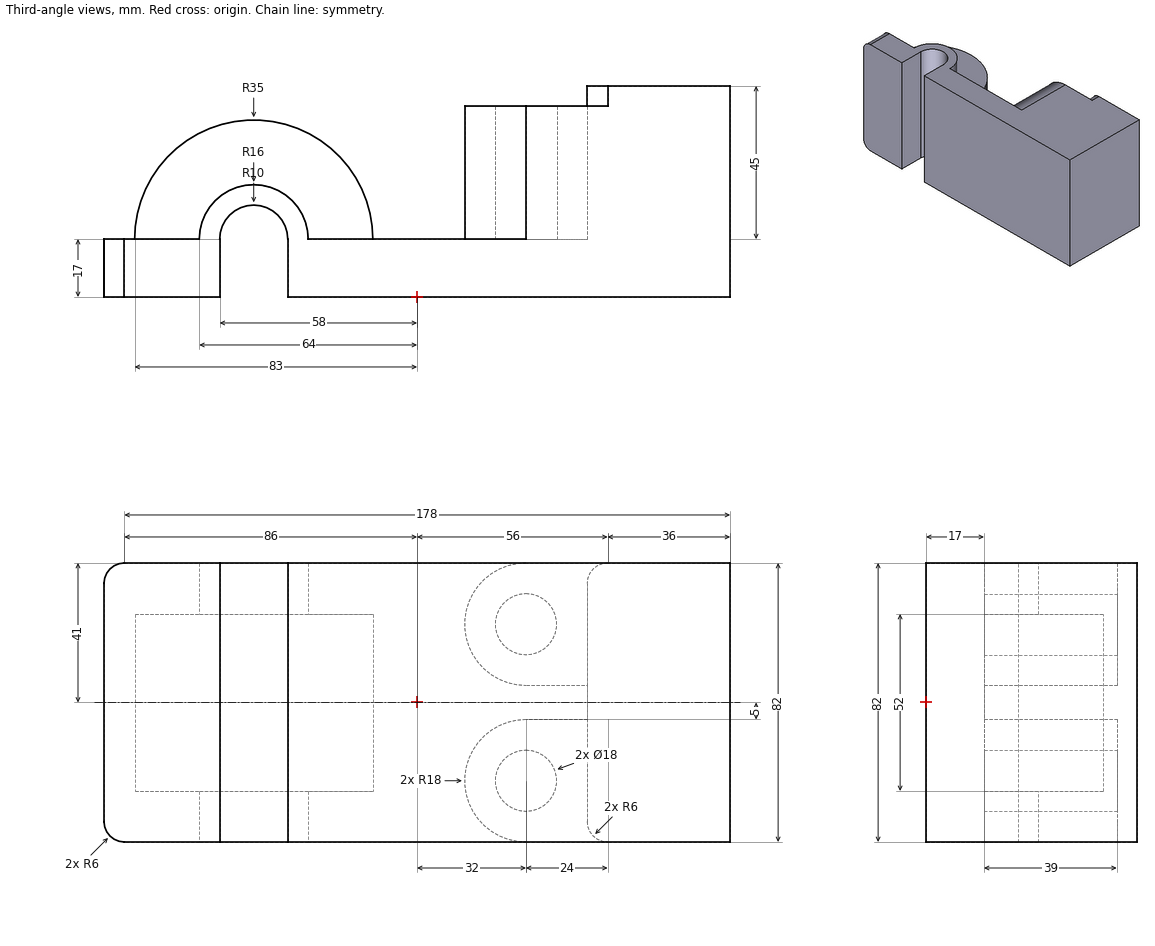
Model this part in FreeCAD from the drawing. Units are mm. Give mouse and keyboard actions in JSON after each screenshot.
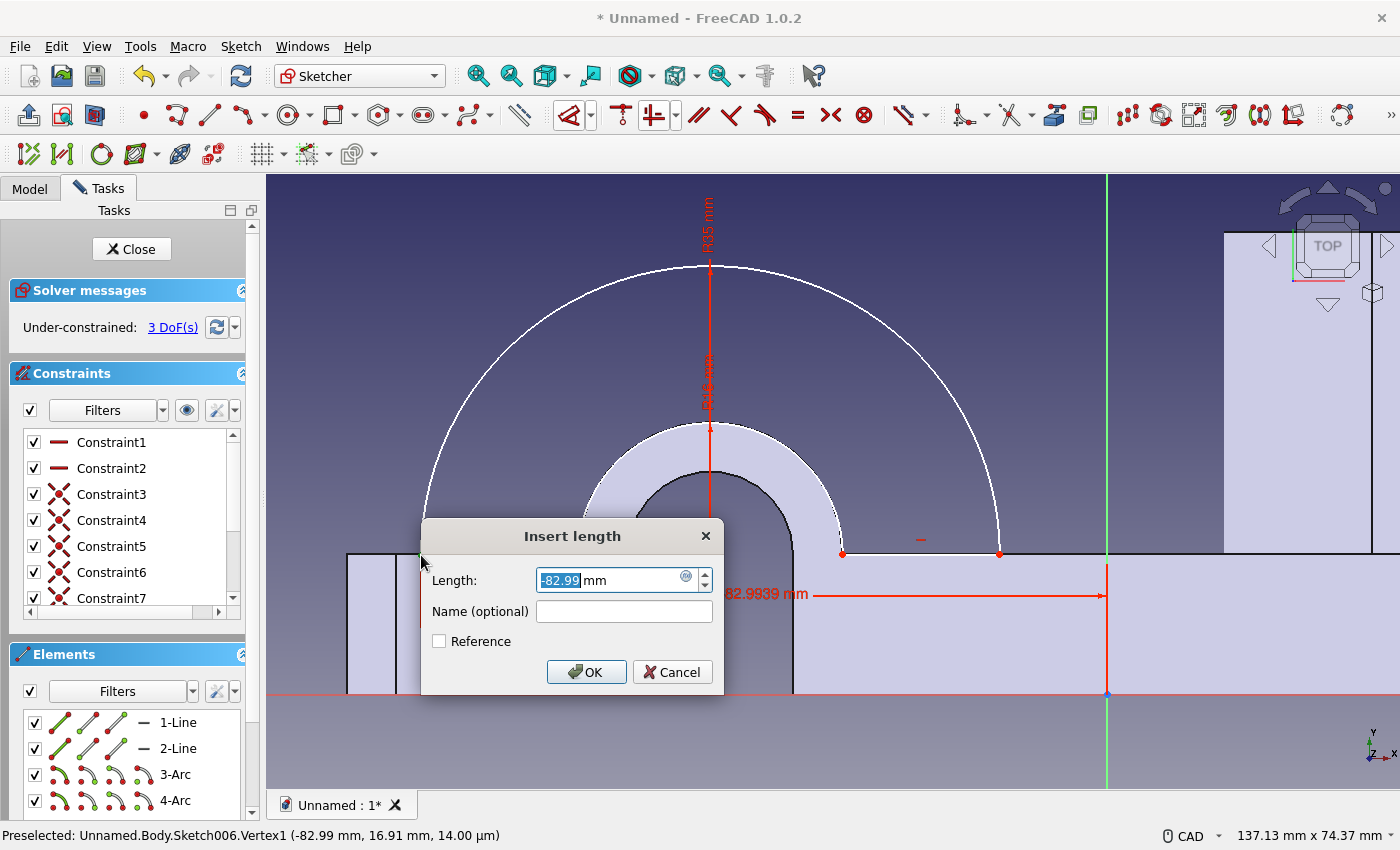
{"action": "type", "text": "-83"}
{"action": "key", "text": "Return"}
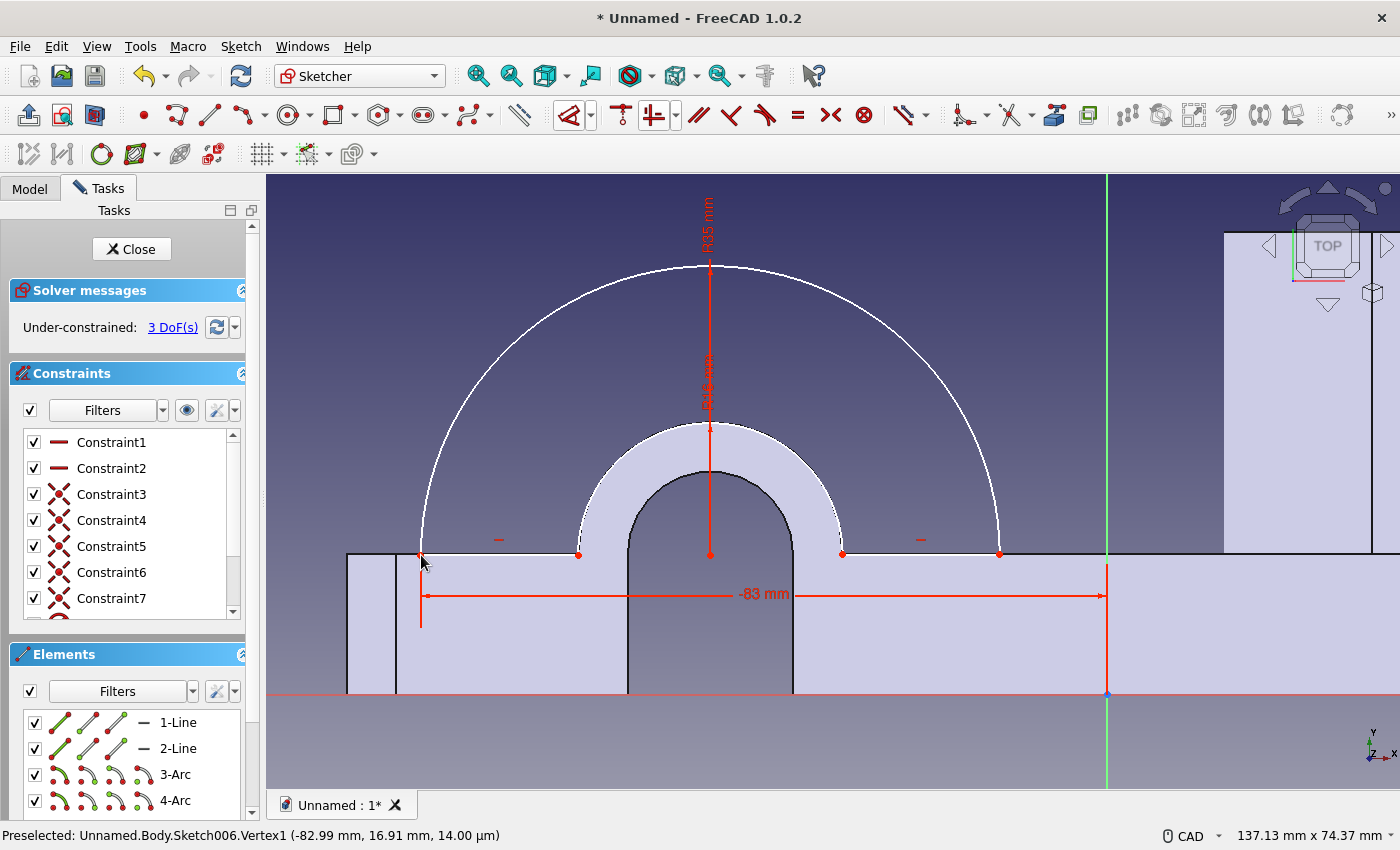
{"action": "left_click", "coordinate": [421, 555]}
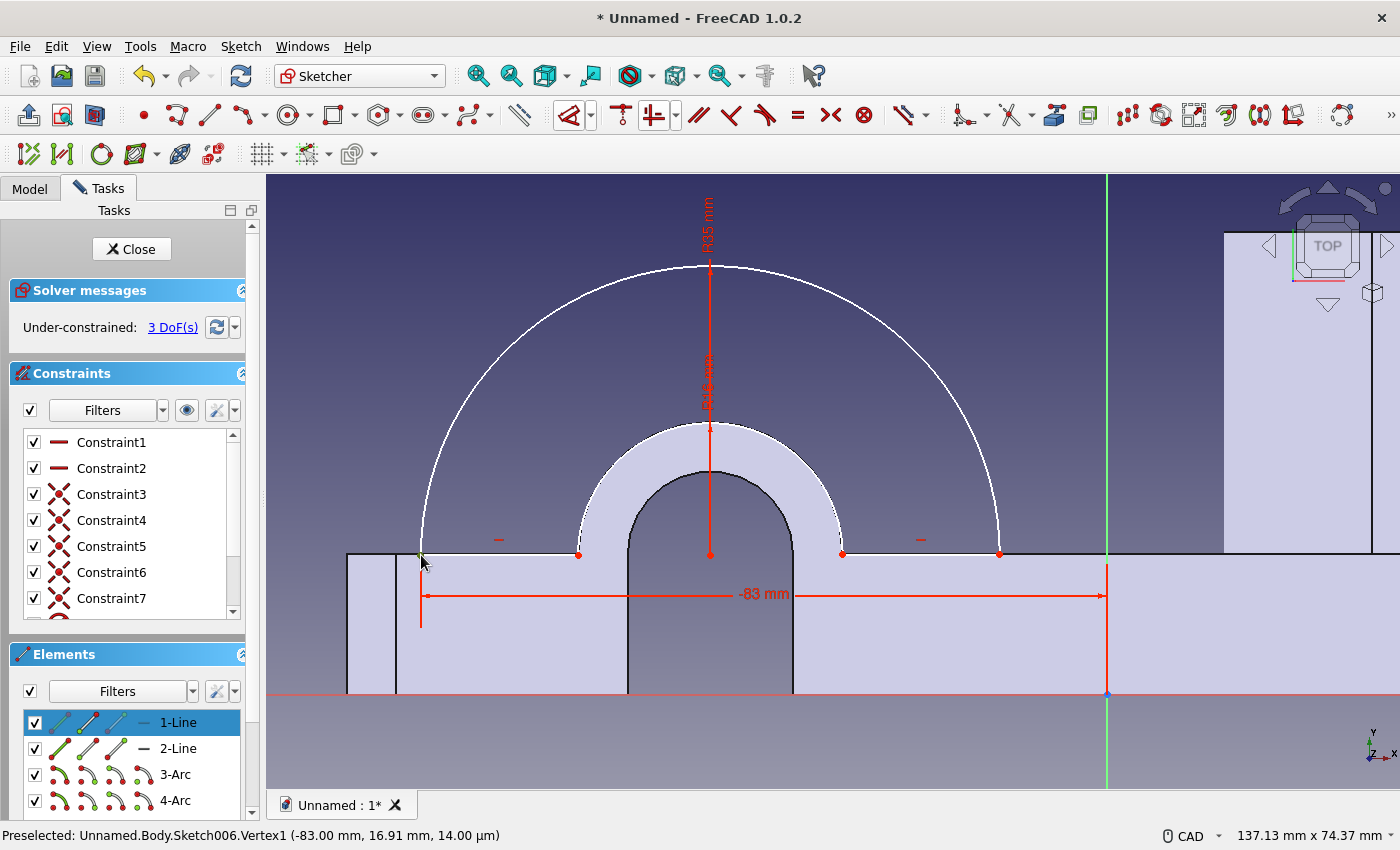
{"action": "left_click", "coordinate": [590, 116]}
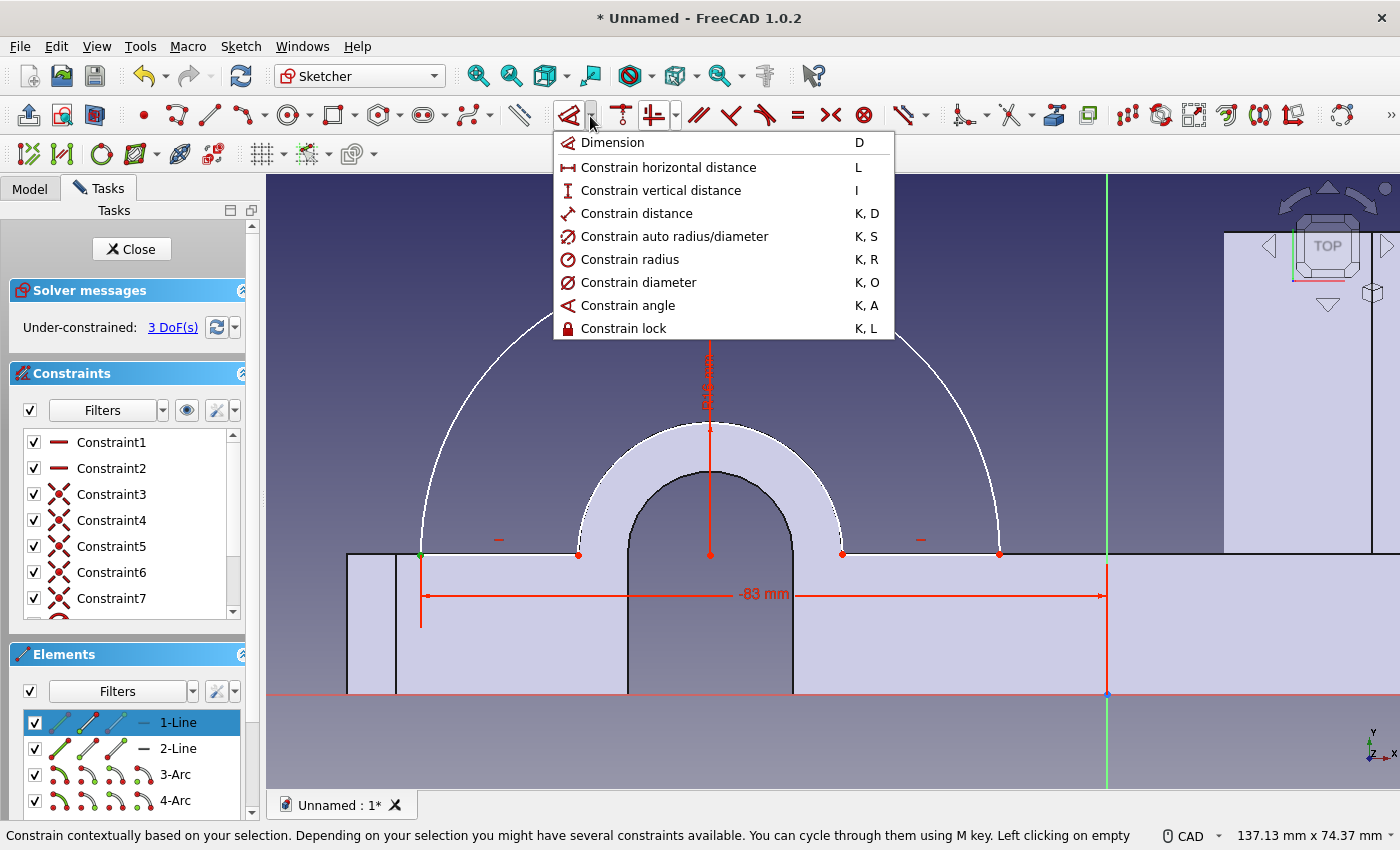
{"action": "left_click", "coordinate": [724, 190]}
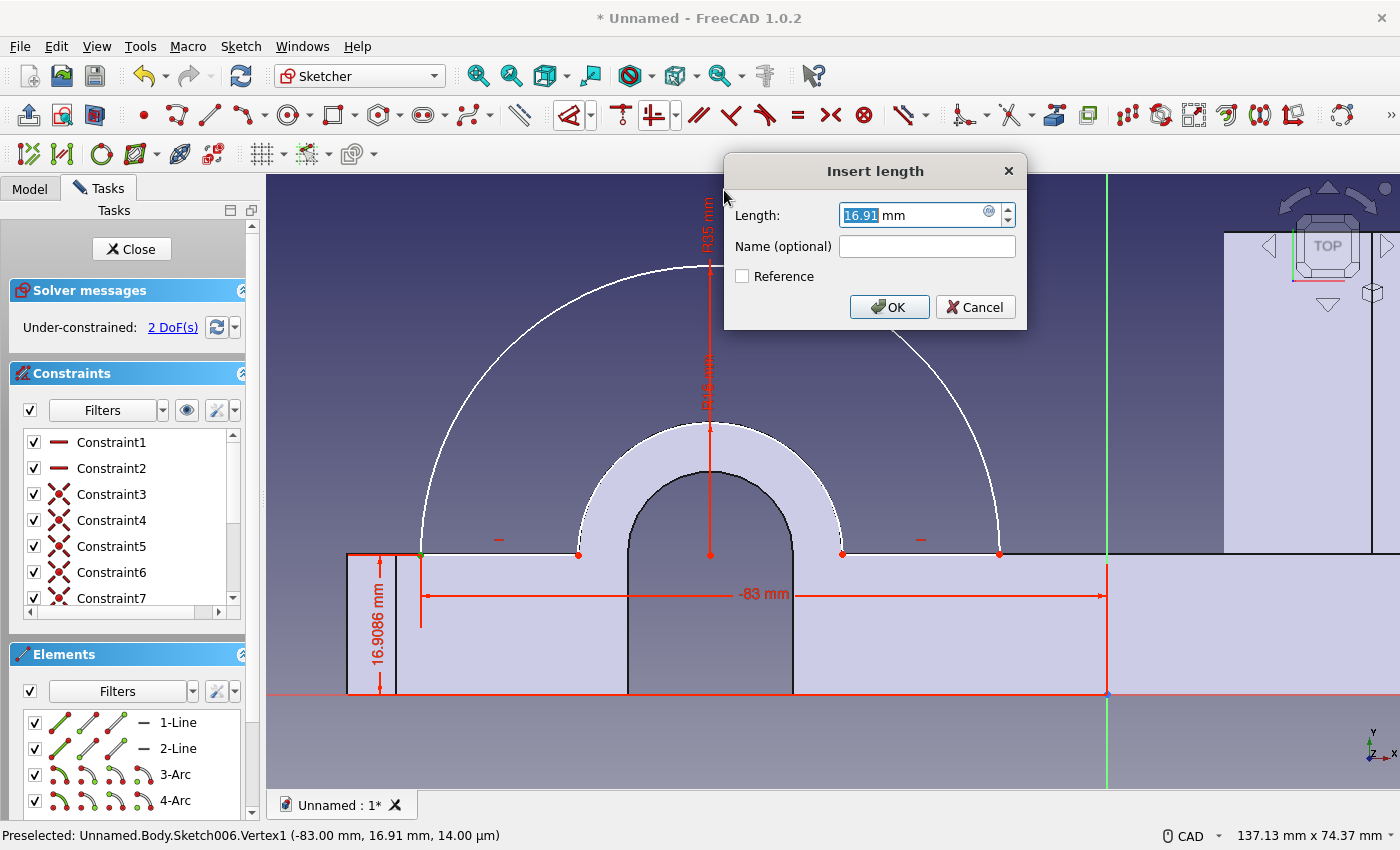
{"action": "type", "text": "17"}
{"action": "key", "text": "Return"}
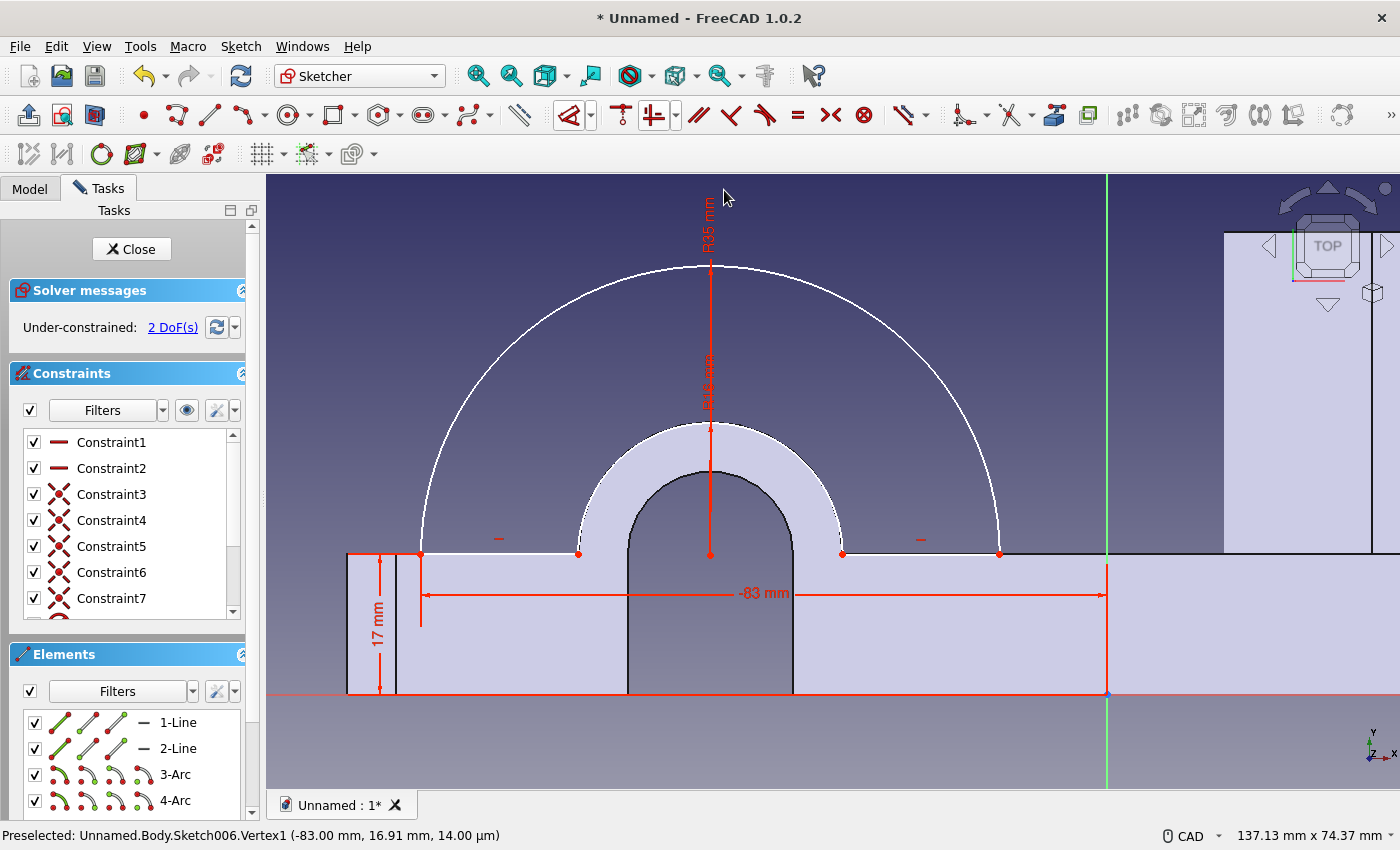
{"action": "left_click", "coordinate": [843, 555]}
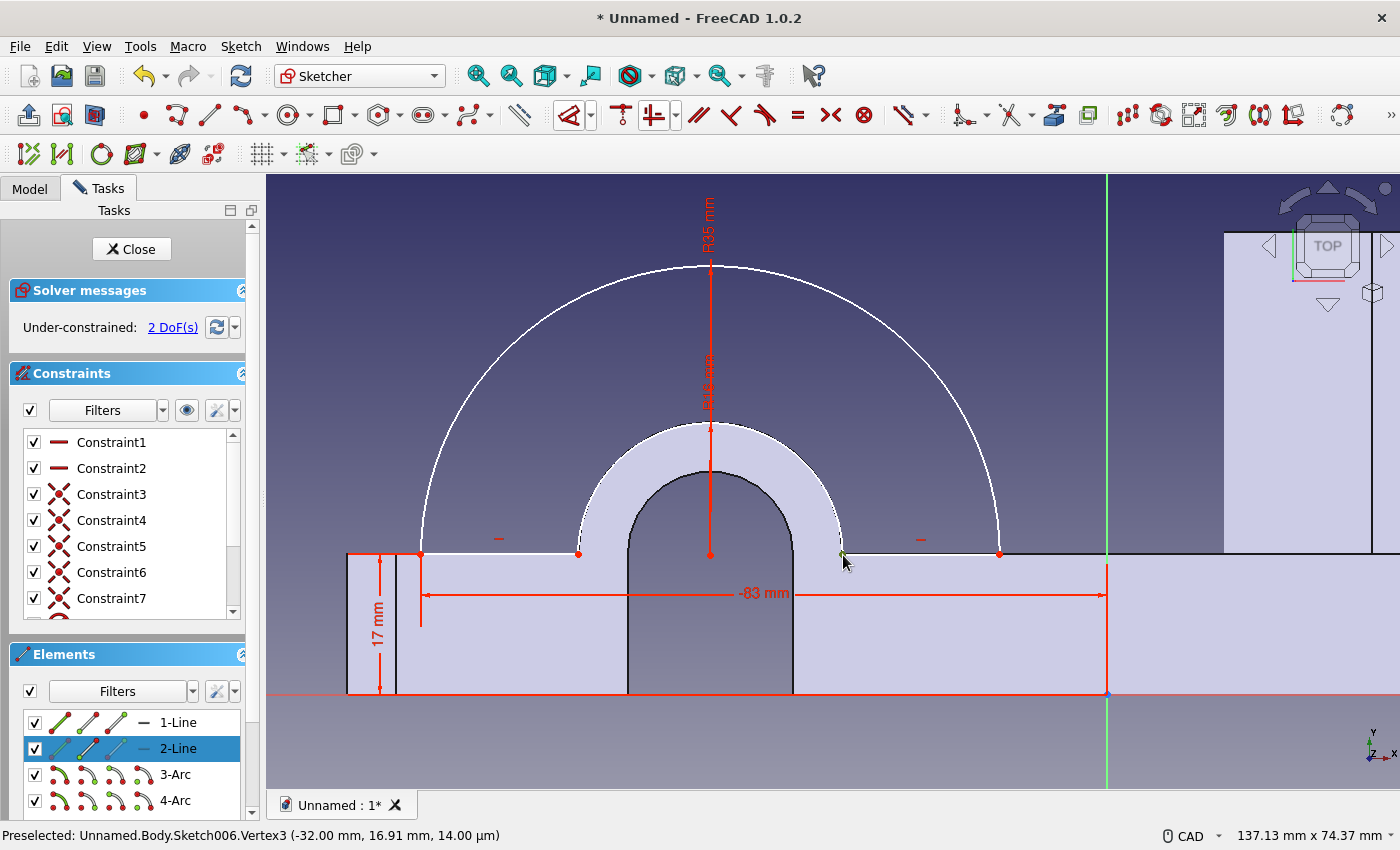
{"action": "left_click", "coordinate": [590, 116]}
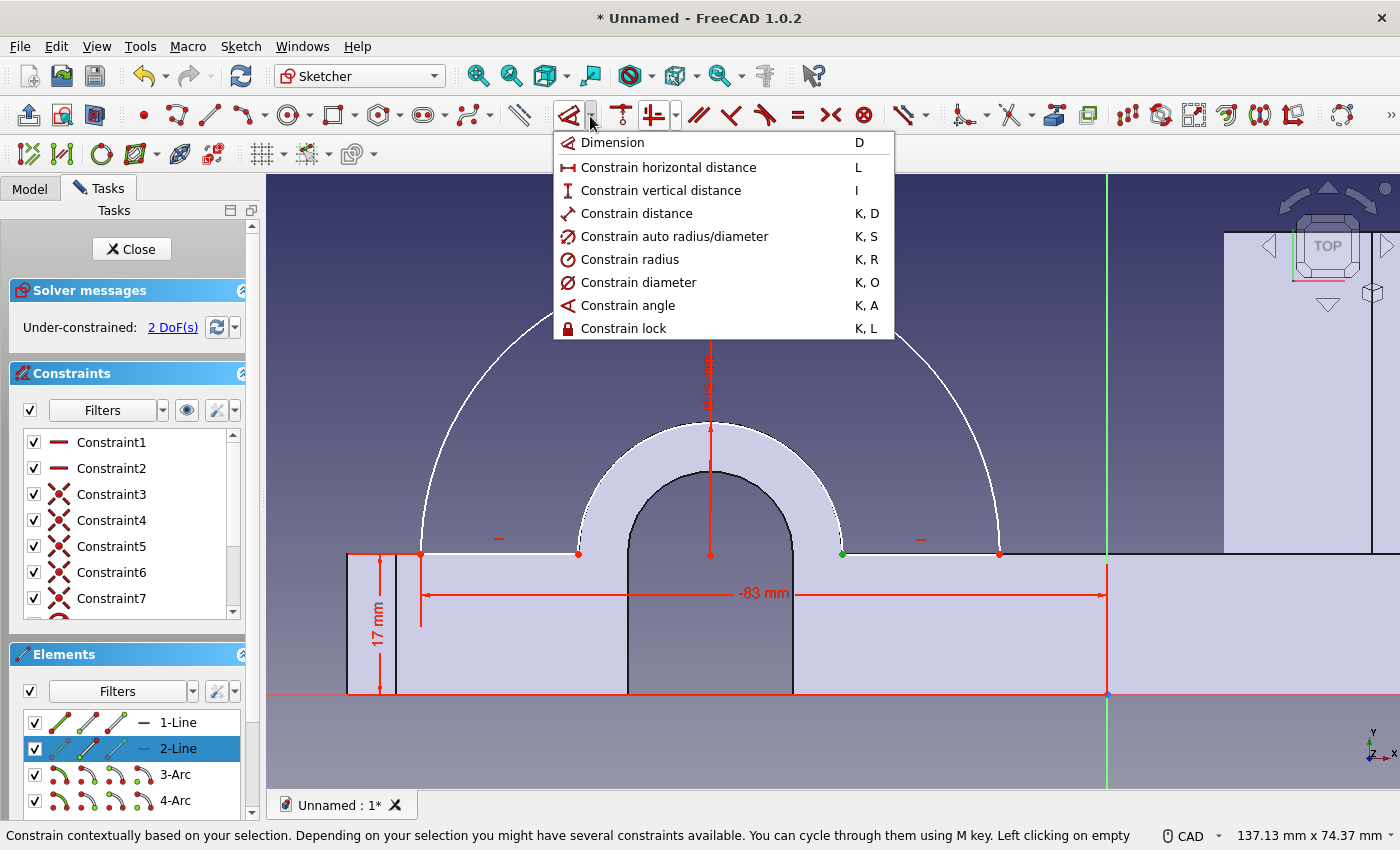
{"action": "left_click", "coordinate": [724, 190]}